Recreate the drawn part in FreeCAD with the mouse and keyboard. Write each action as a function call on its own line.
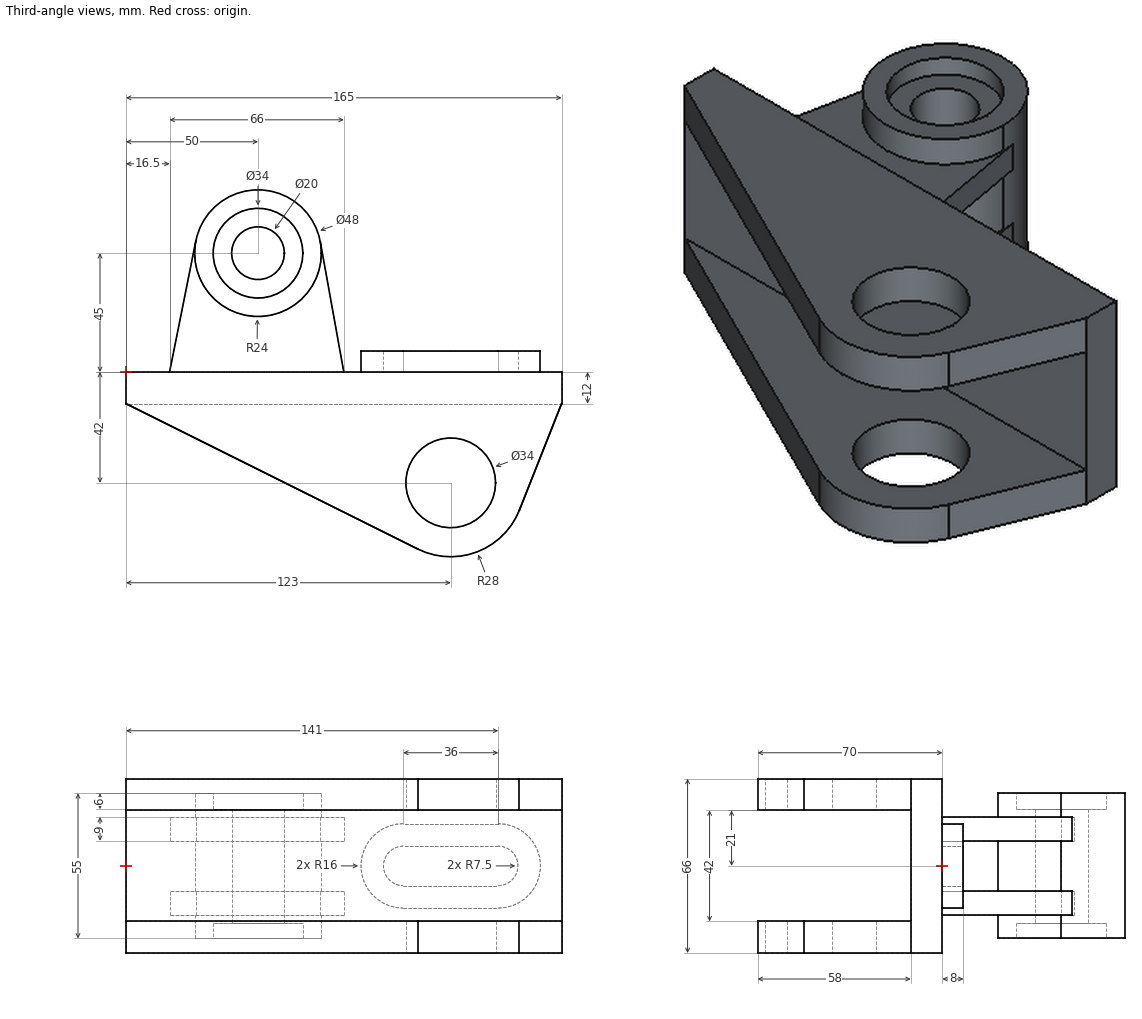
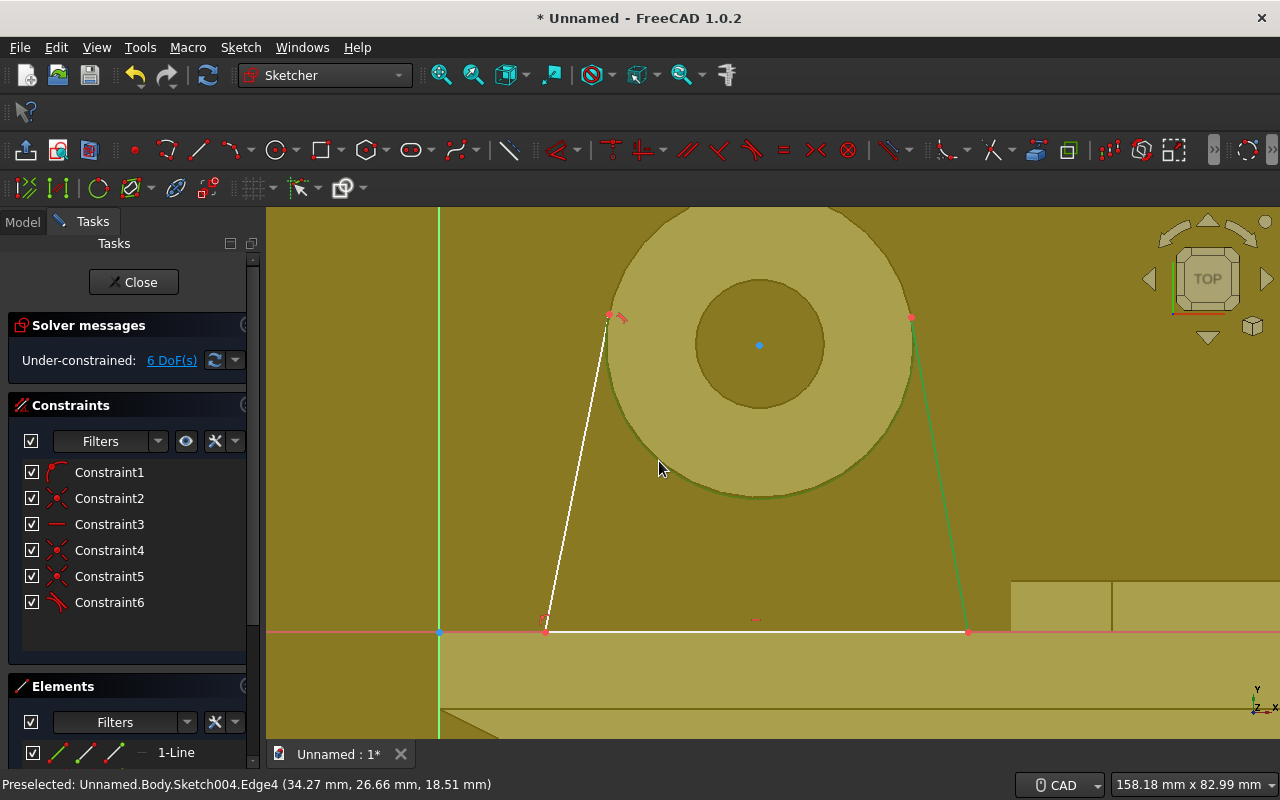
key(t)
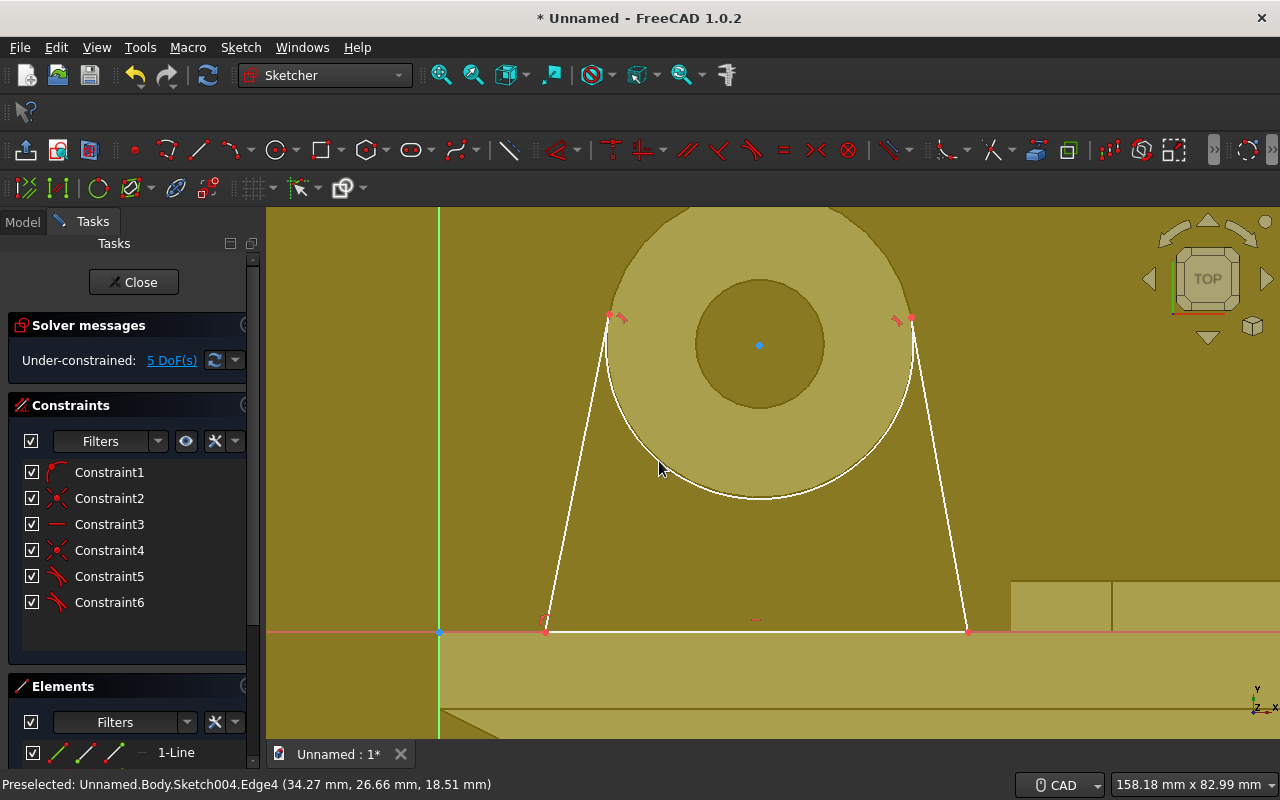
key(d)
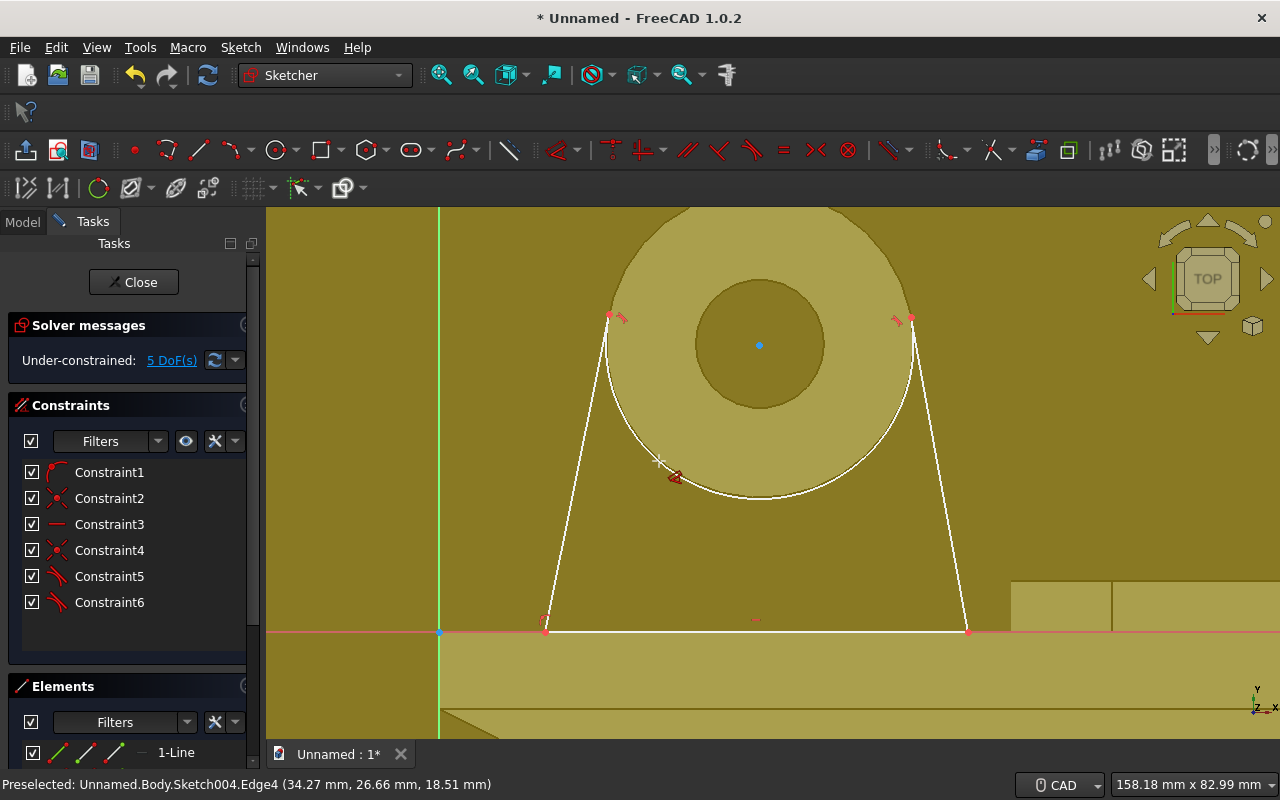
click(659, 462)
click(638, 486)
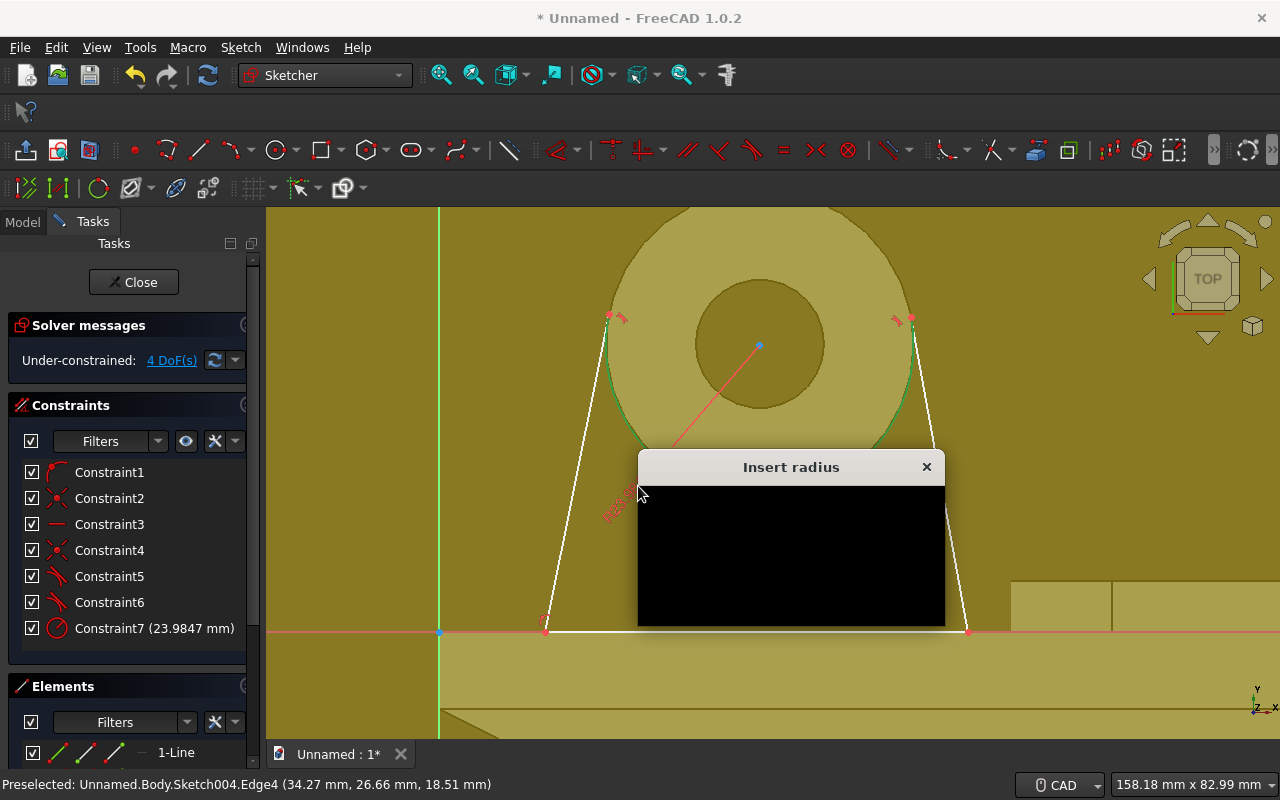
text(24)
key(Return)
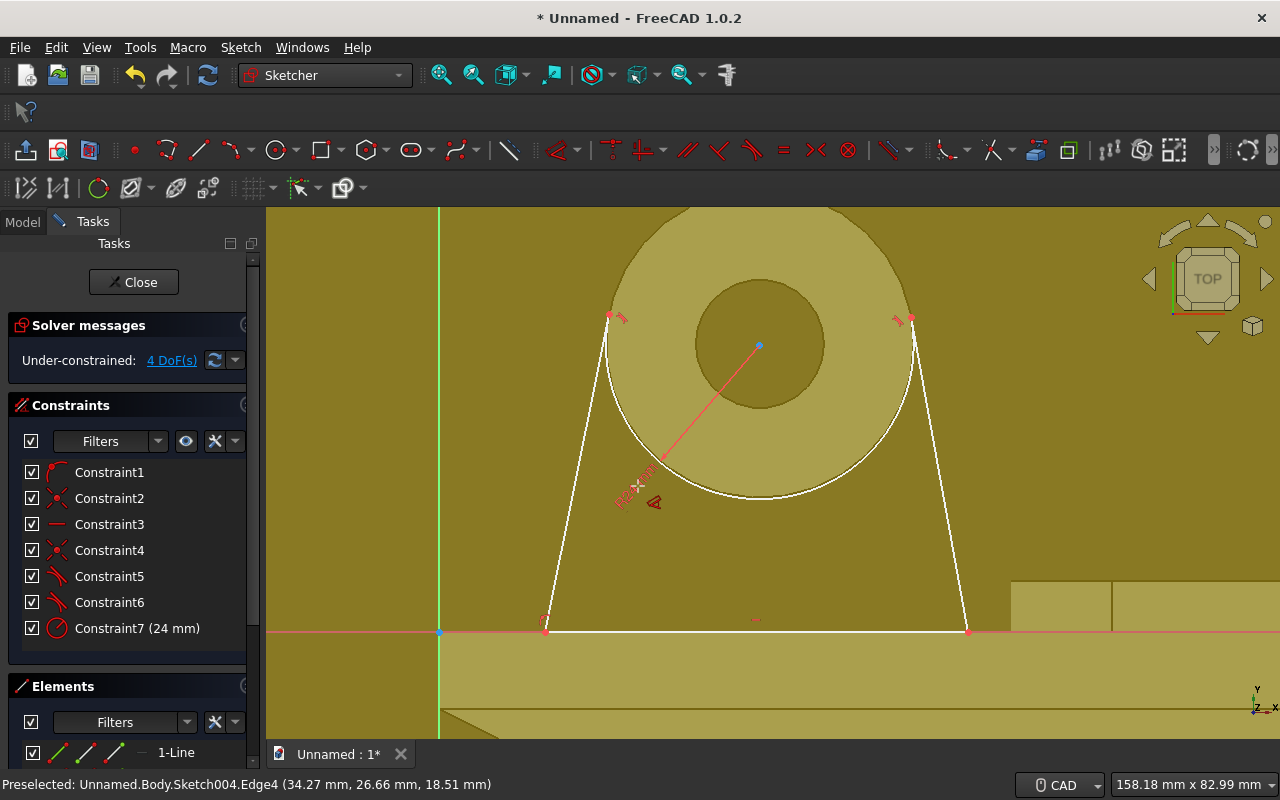
click(672, 632)
click(756, 666)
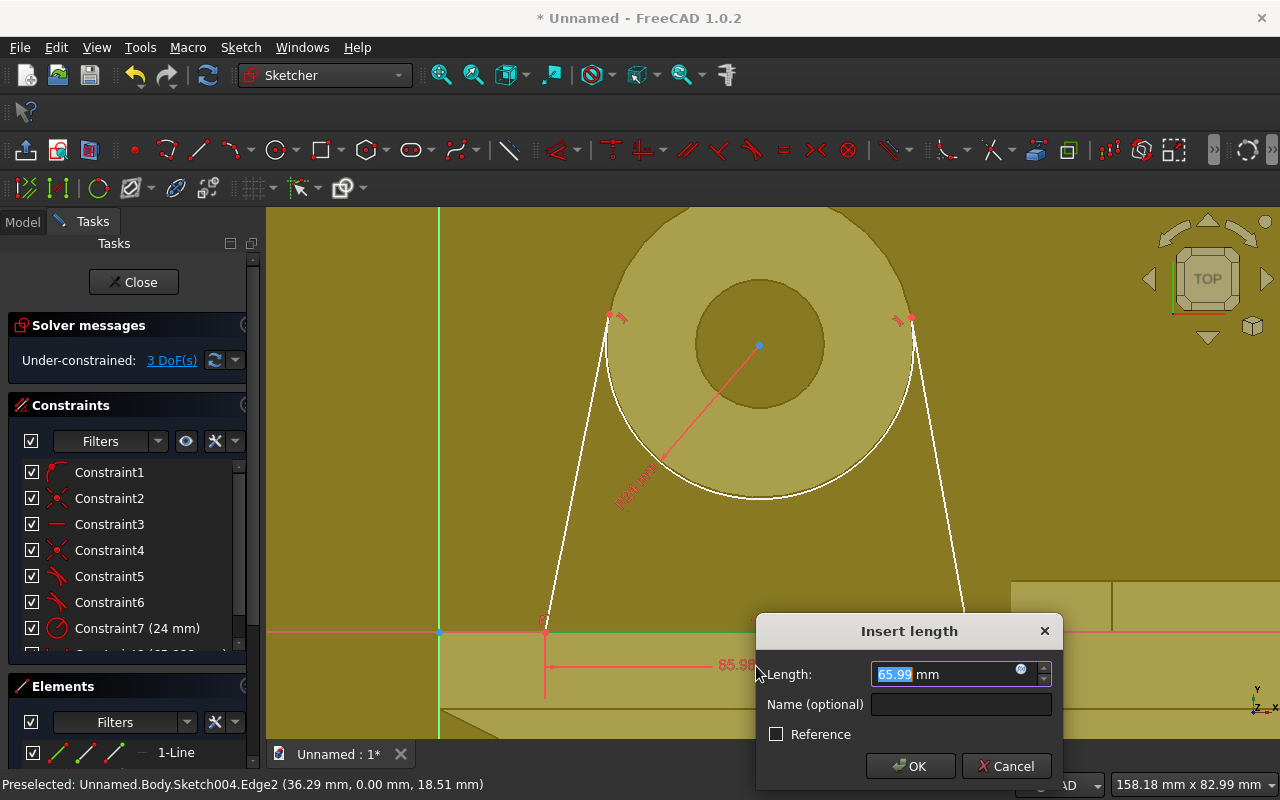
text(66)
key(Return)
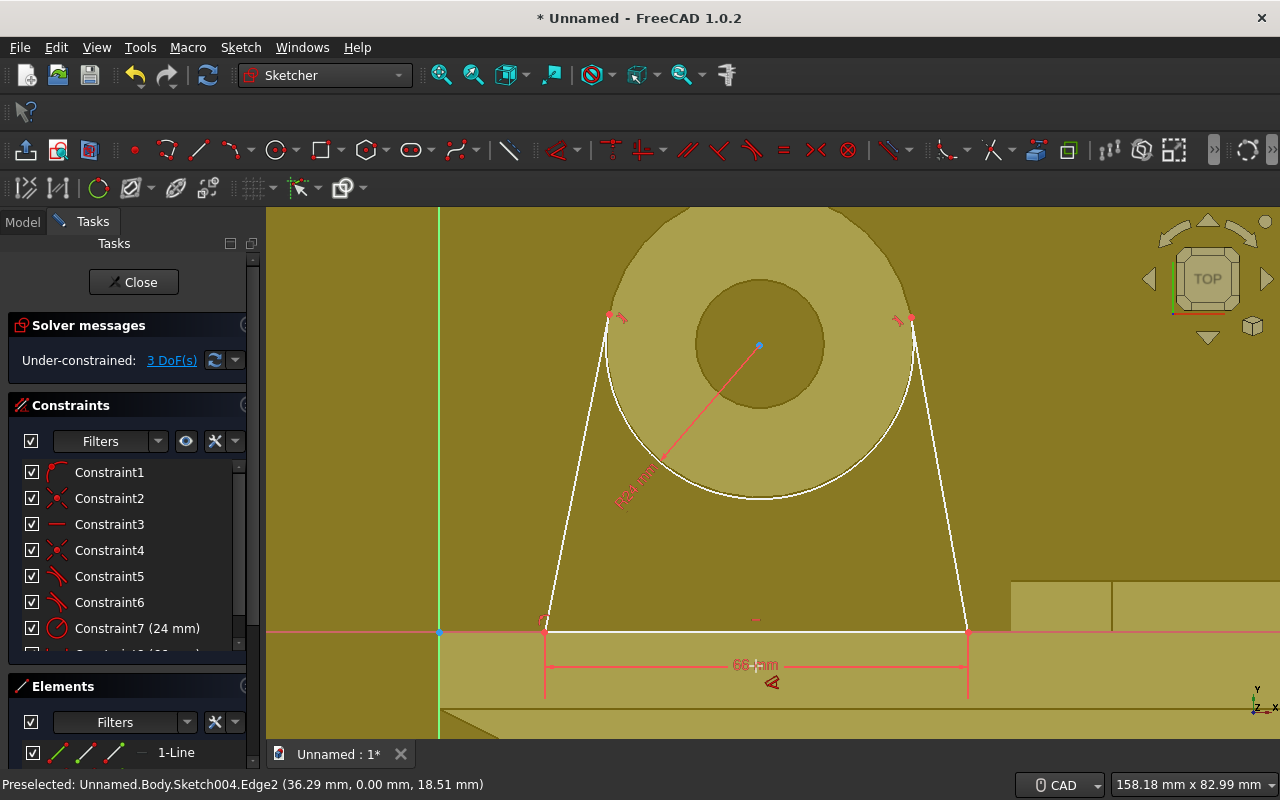
click(760, 345)
click(600, 666)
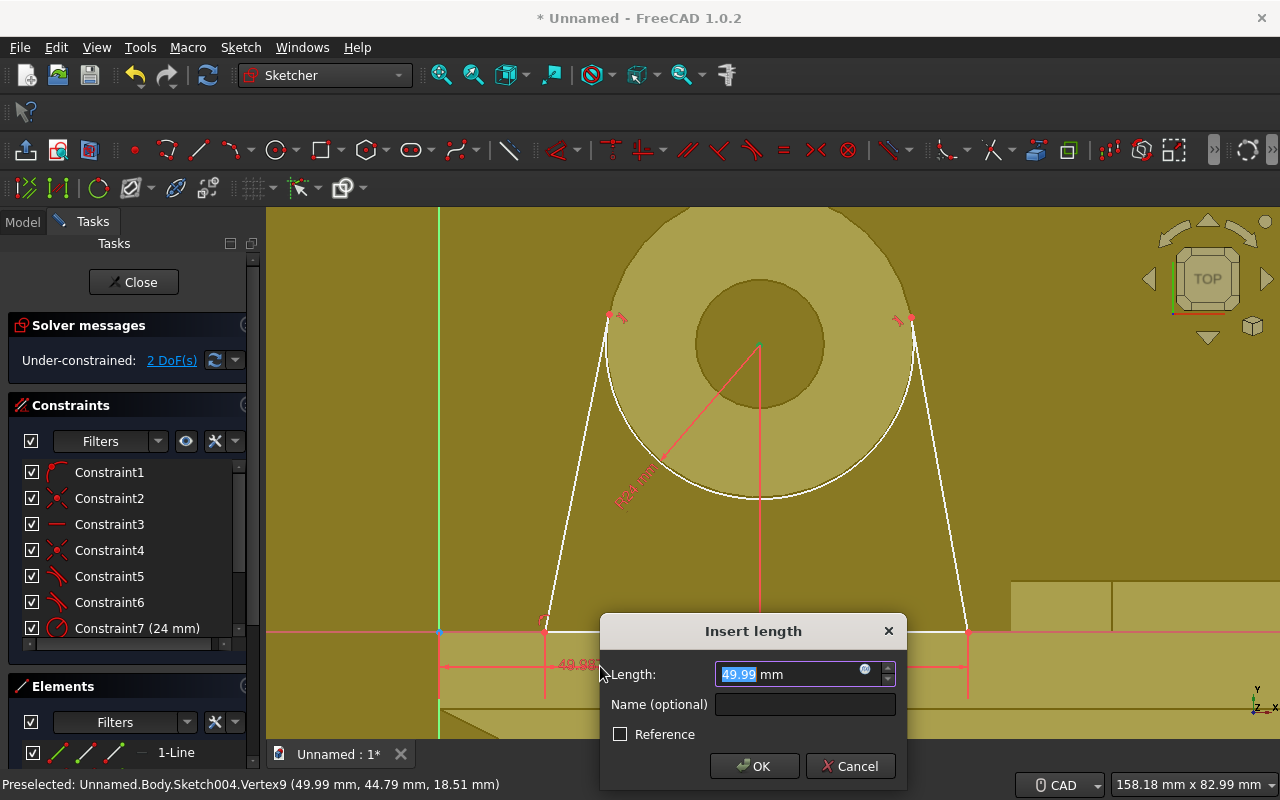
text(50)
key(Return)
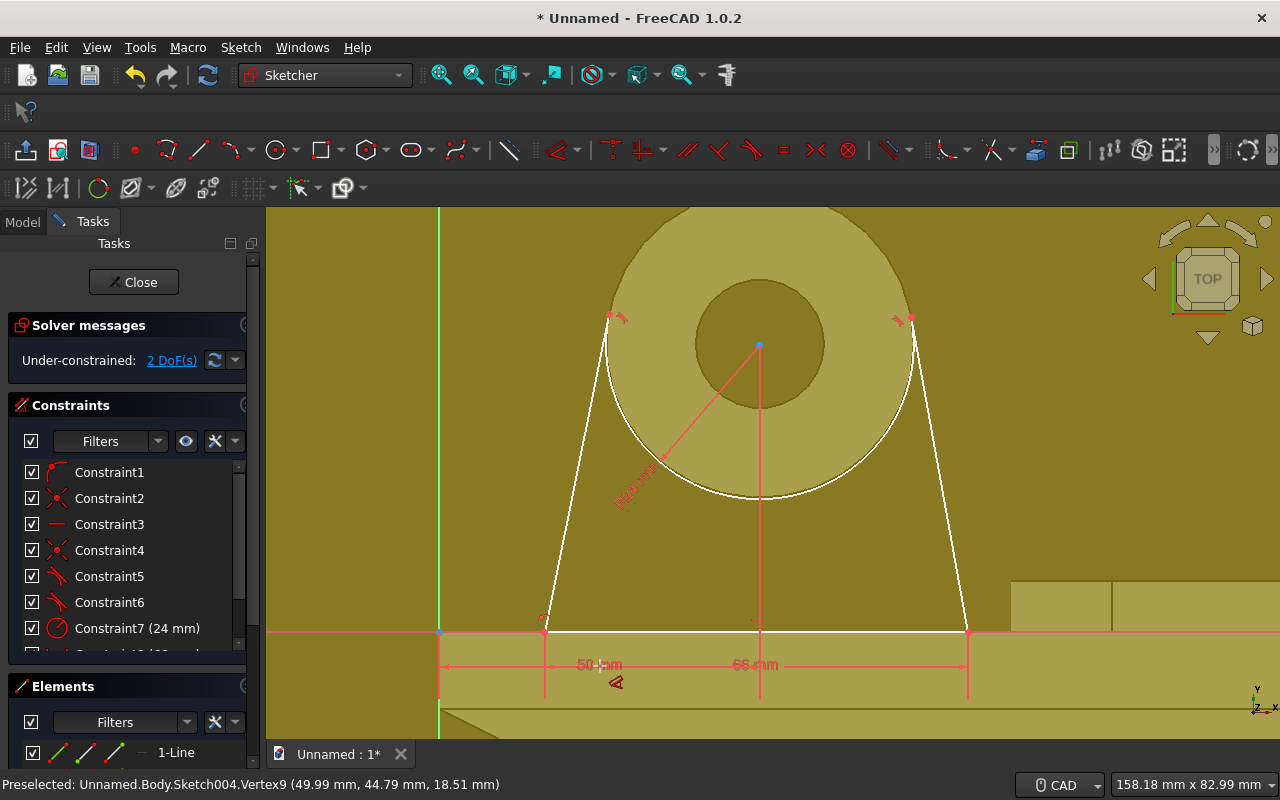
click(760, 345)
click(405, 489)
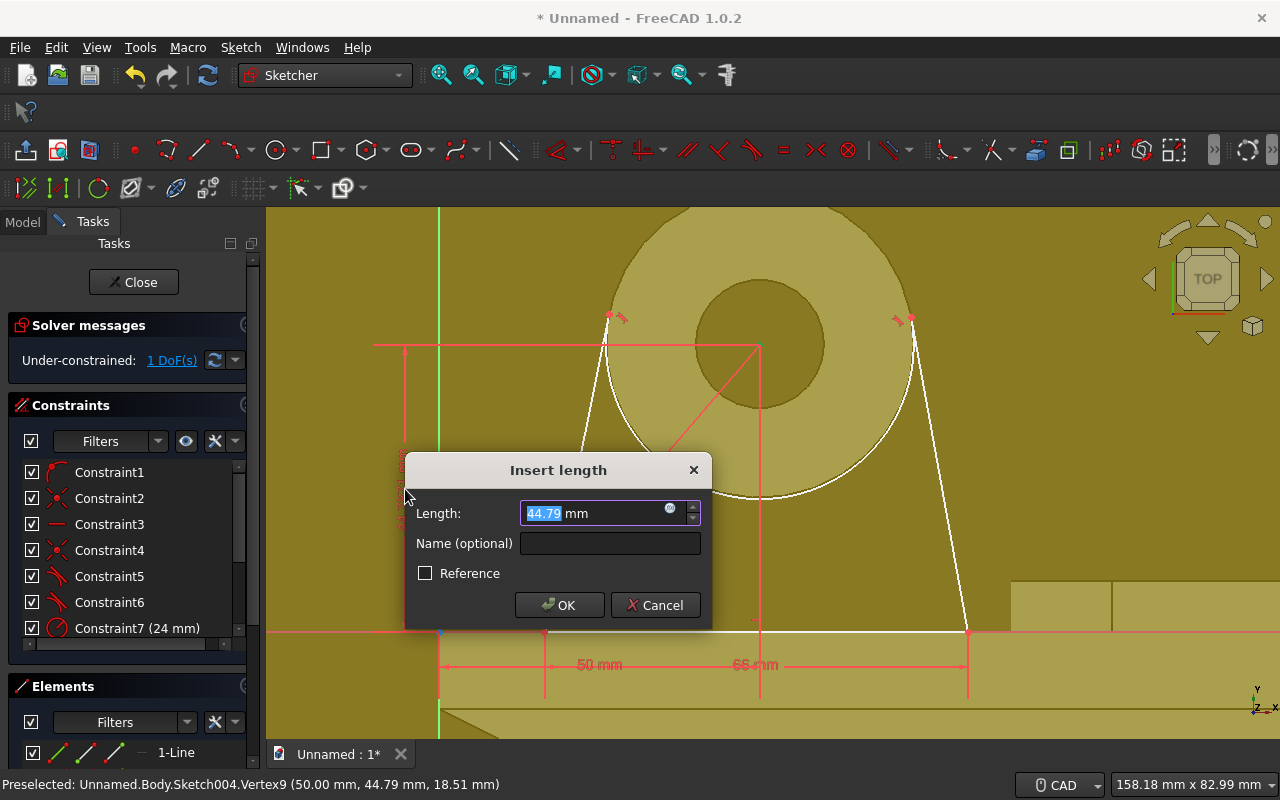
text(45)
key(Return)